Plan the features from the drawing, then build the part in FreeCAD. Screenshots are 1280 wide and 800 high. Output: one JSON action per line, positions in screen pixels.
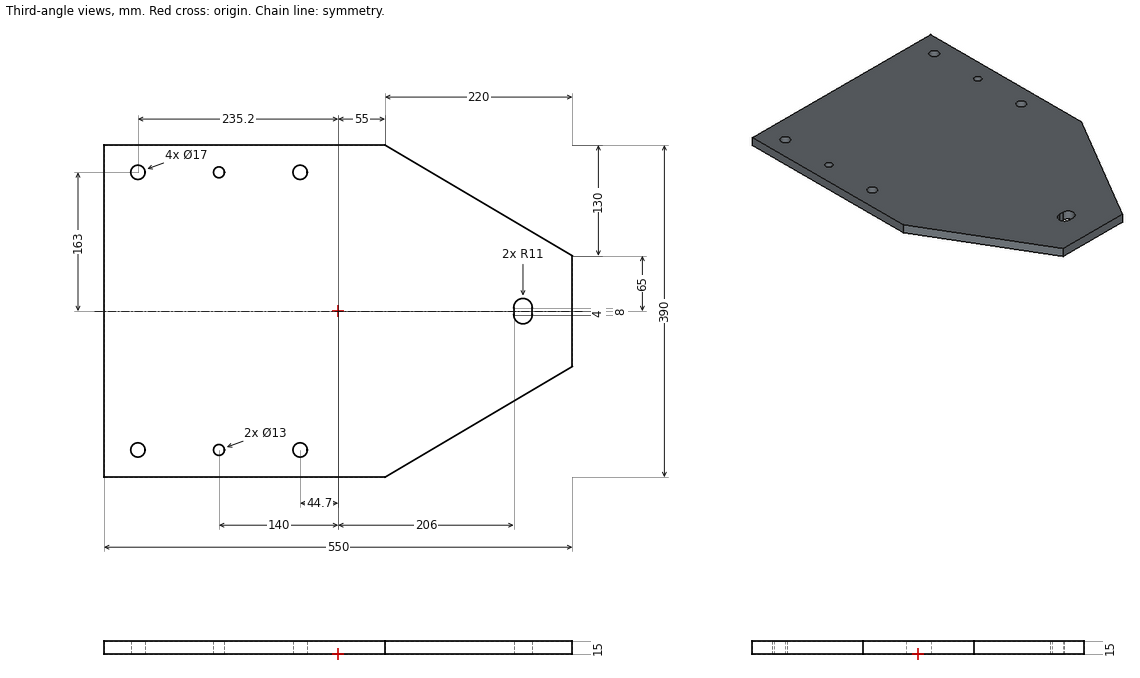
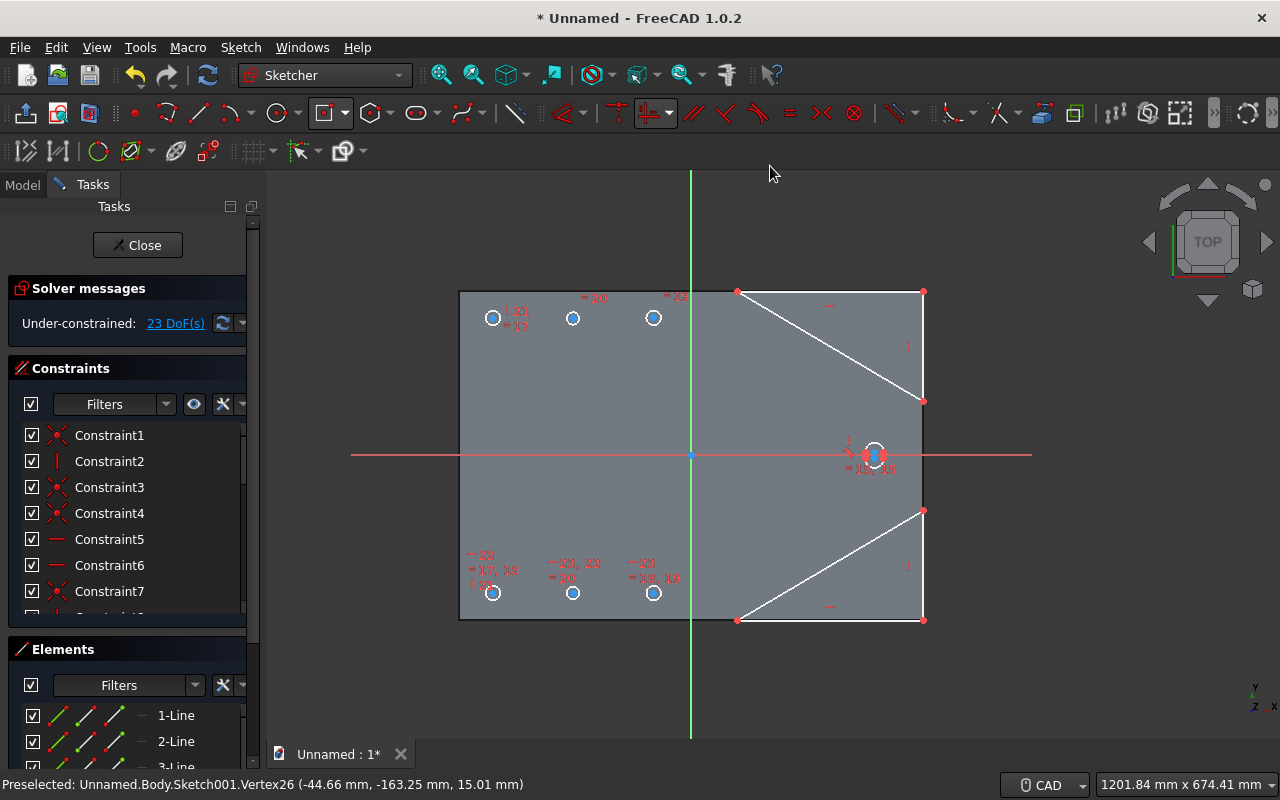
{"action": "left_click", "coordinate": [573, 593]}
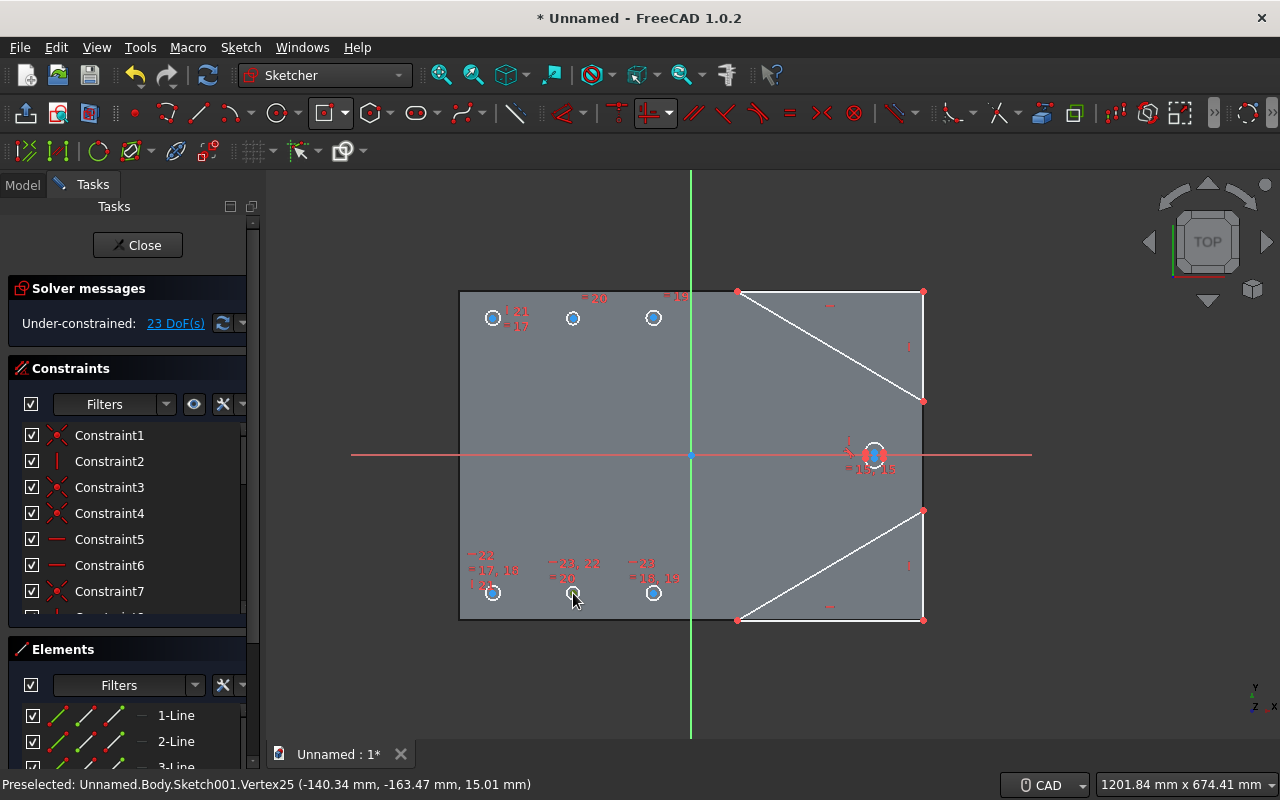
{"action": "left_click", "coordinate": [573, 318]}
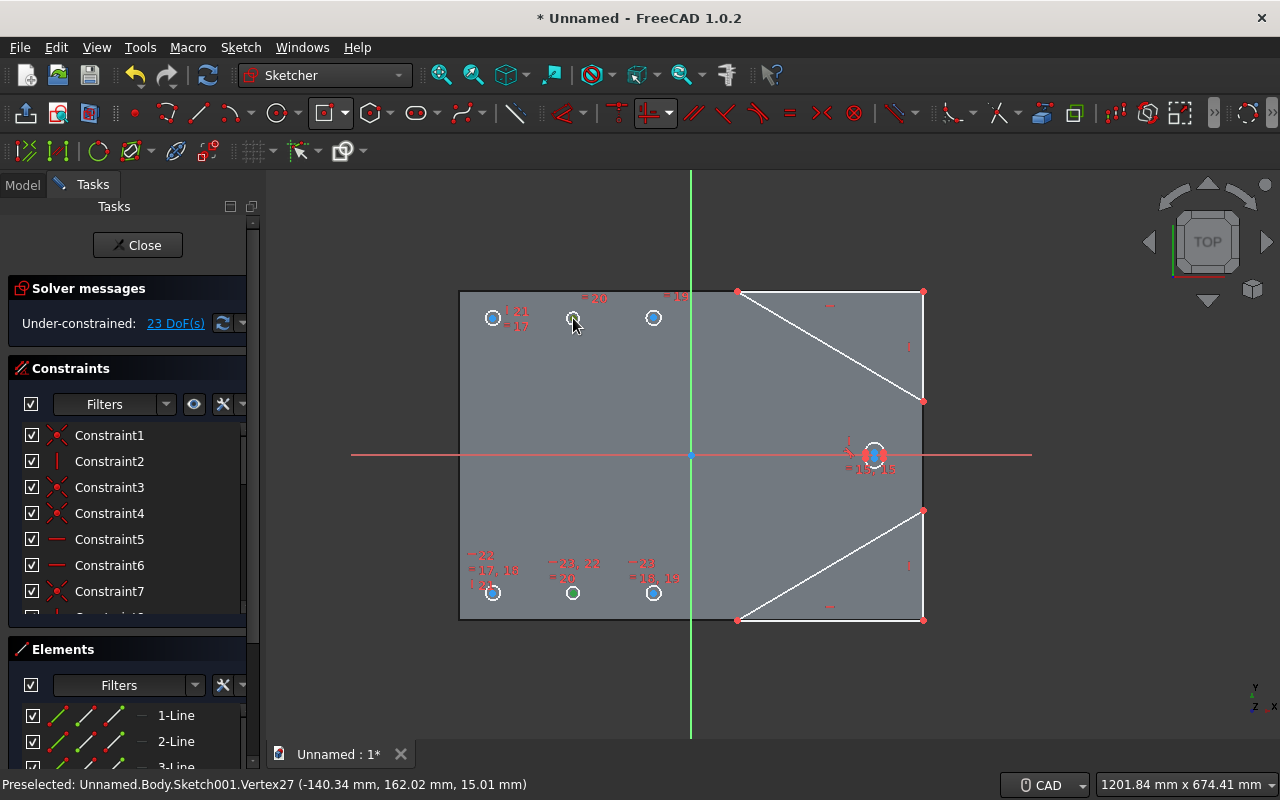
{"action": "left_click", "coordinate": [672, 114]}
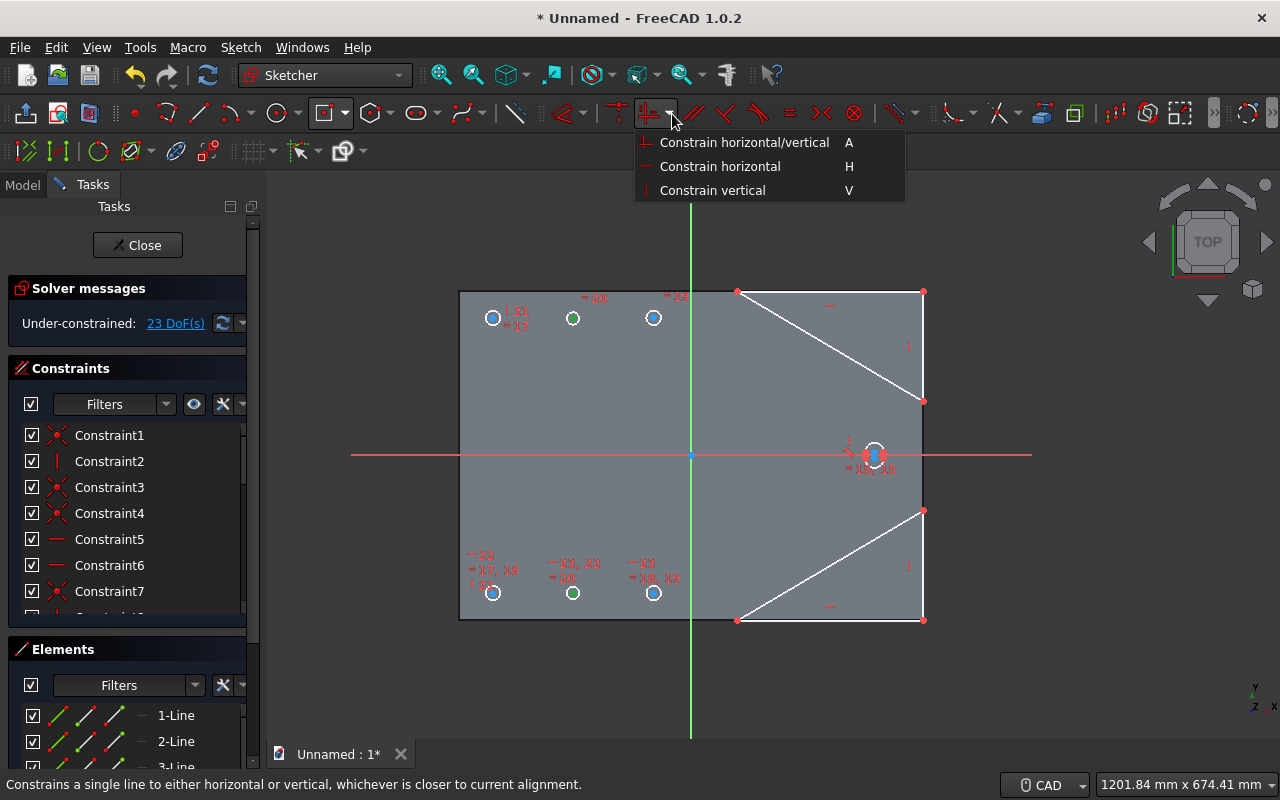
{"action": "left_click", "coordinate": [770, 190]}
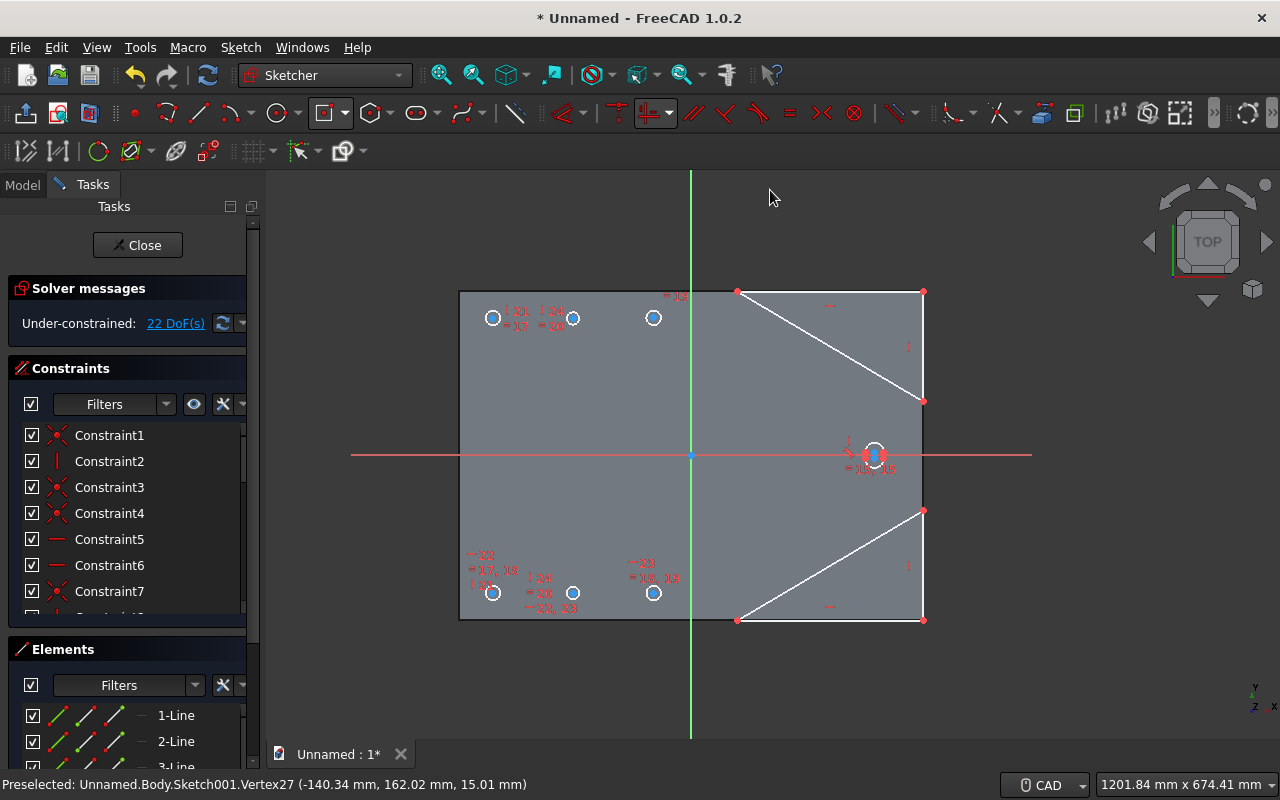
{"action": "left_click", "coordinate": [493, 318]}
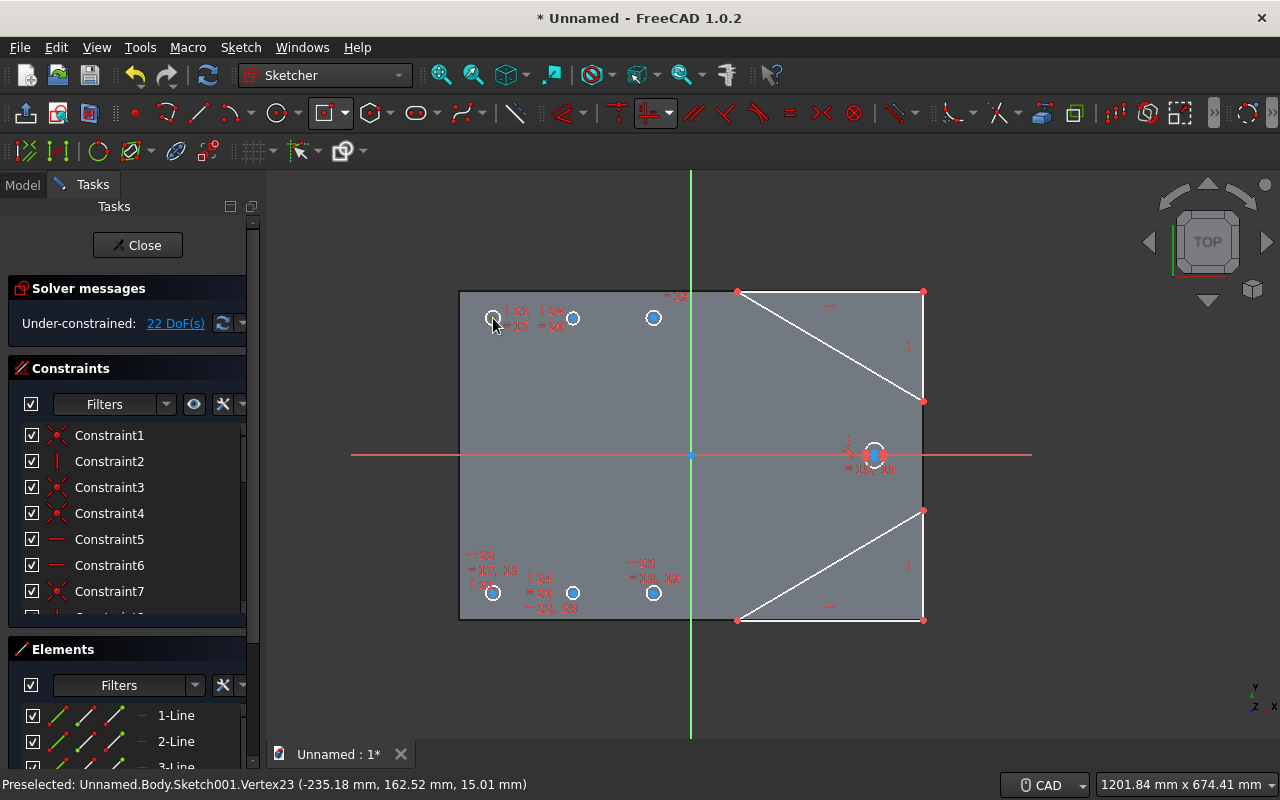
{"action": "left_click", "coordinate": [573, 318]}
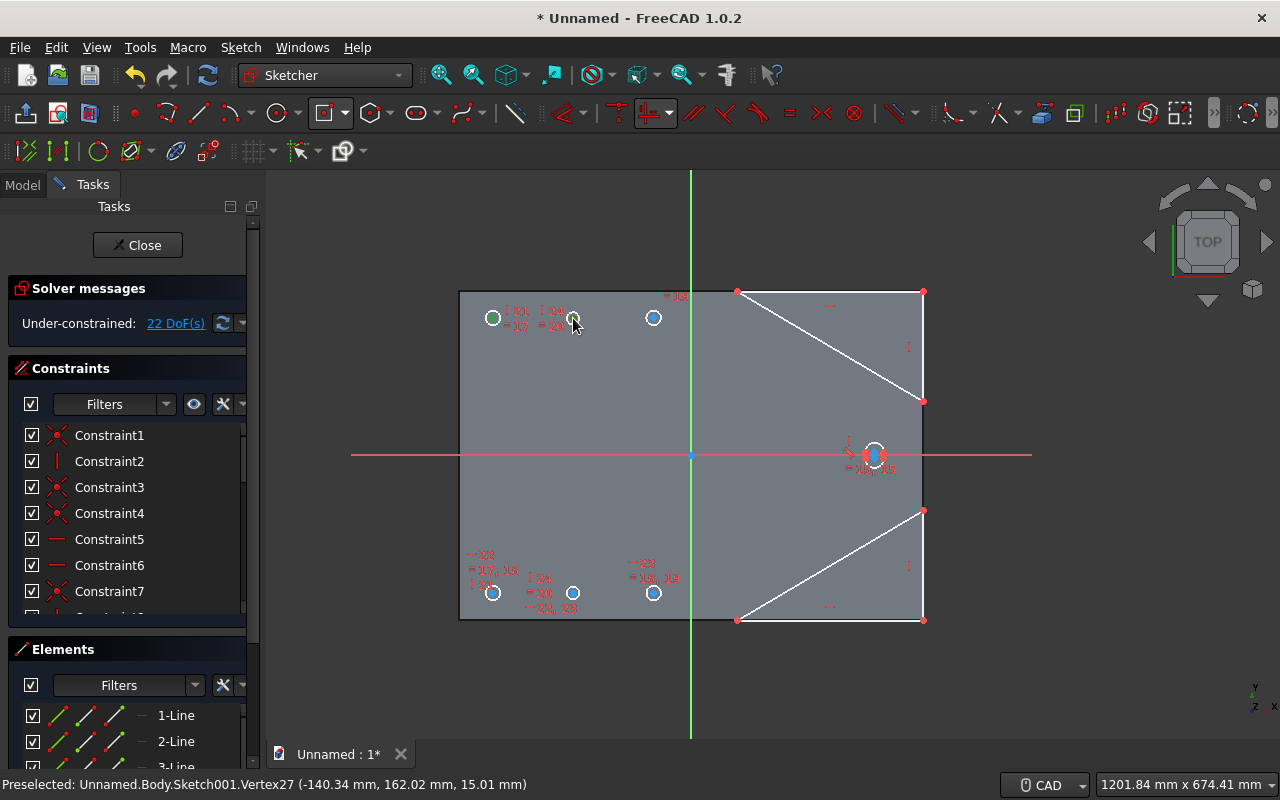
{"action": "key", "text": "h"}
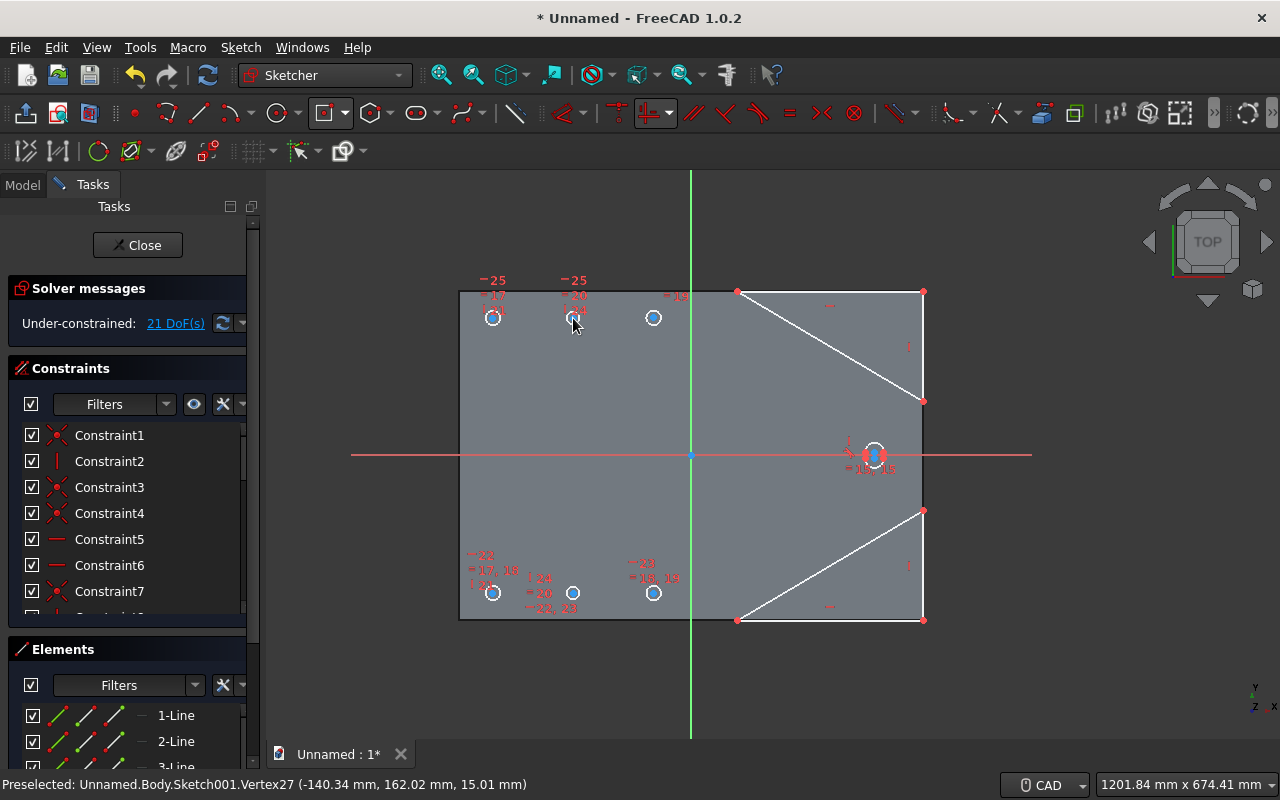
{"action": "left_click", "coordinate": [573, 318]}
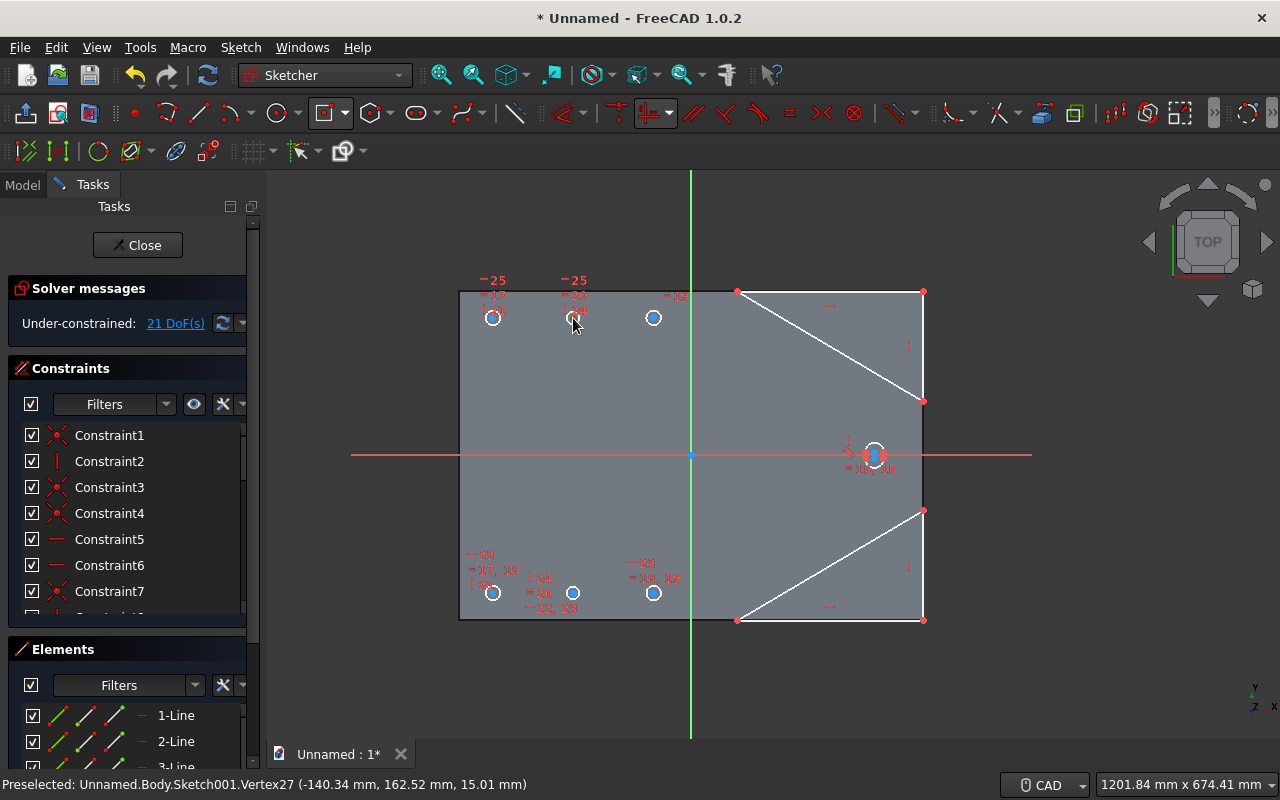
{"action": "left_click", "coordinate": [654, 318]}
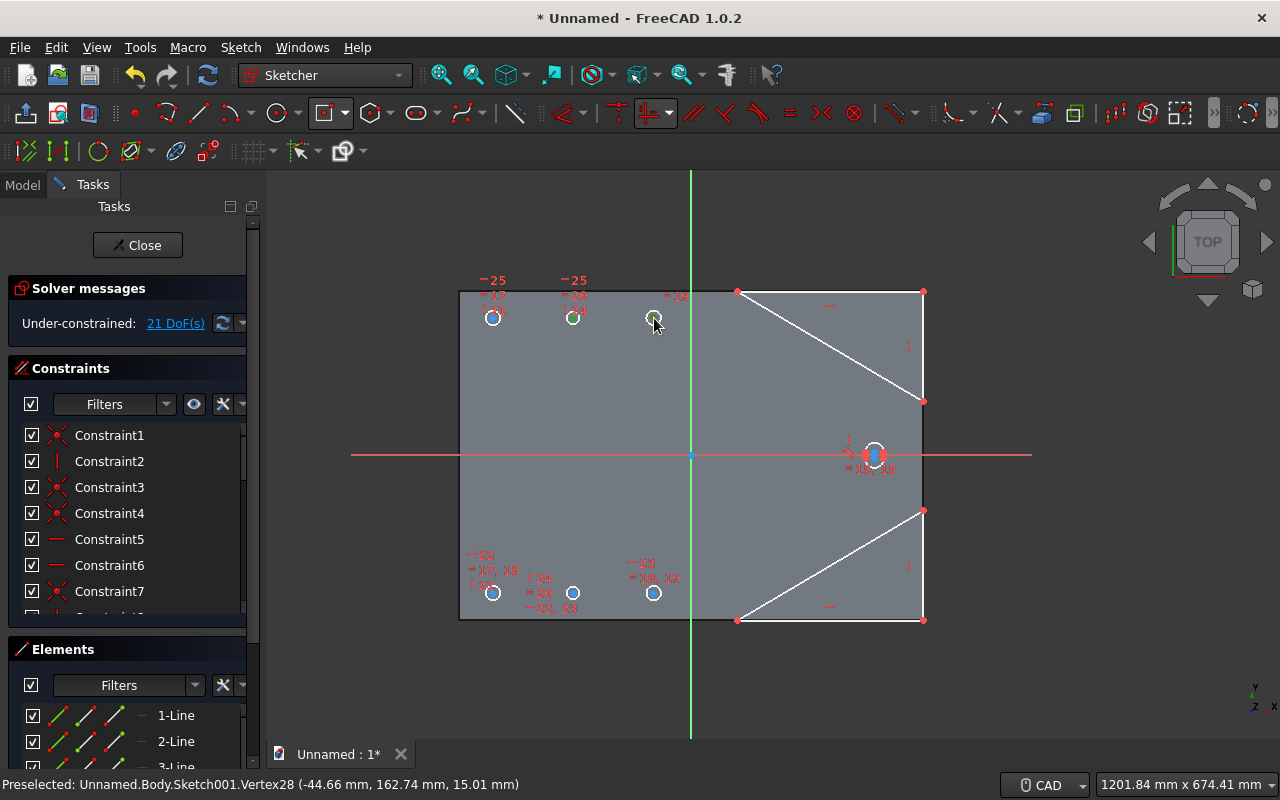
{"action": "key", "text": "h"}